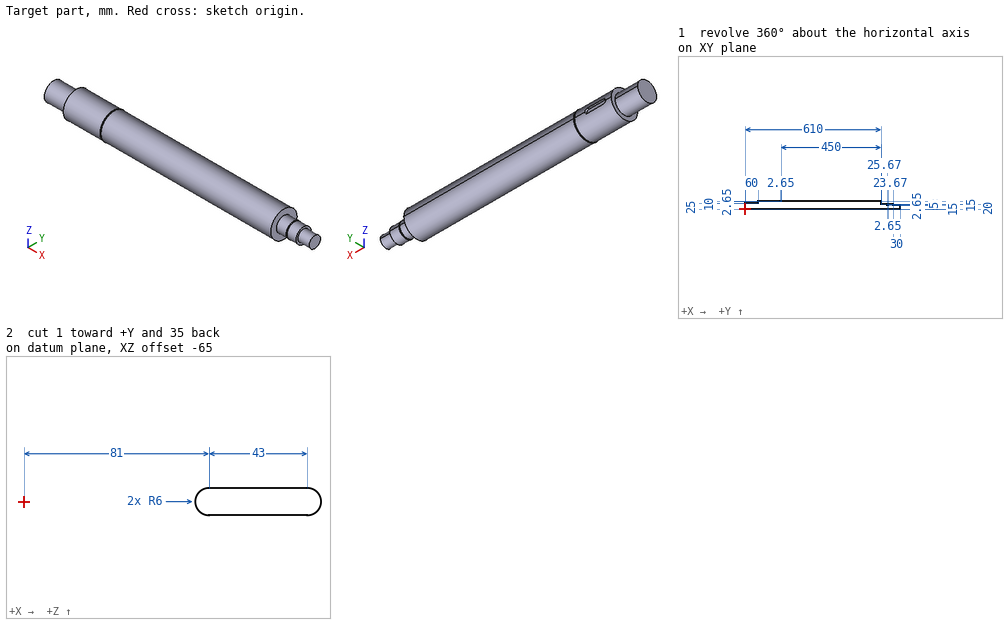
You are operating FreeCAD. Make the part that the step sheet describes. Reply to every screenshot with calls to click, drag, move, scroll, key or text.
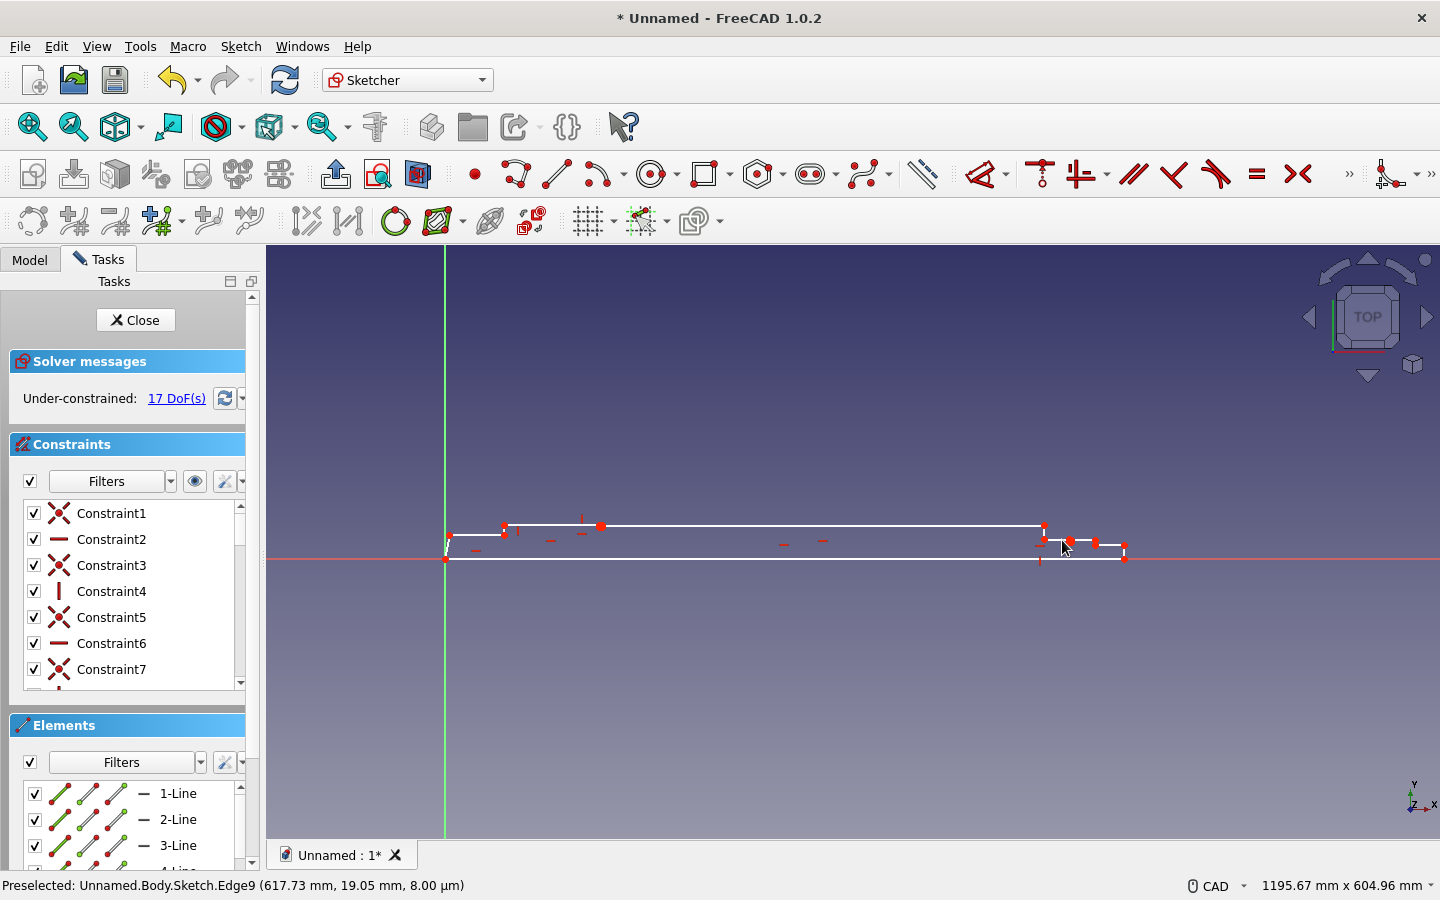
scroll(446, 552, up, 4)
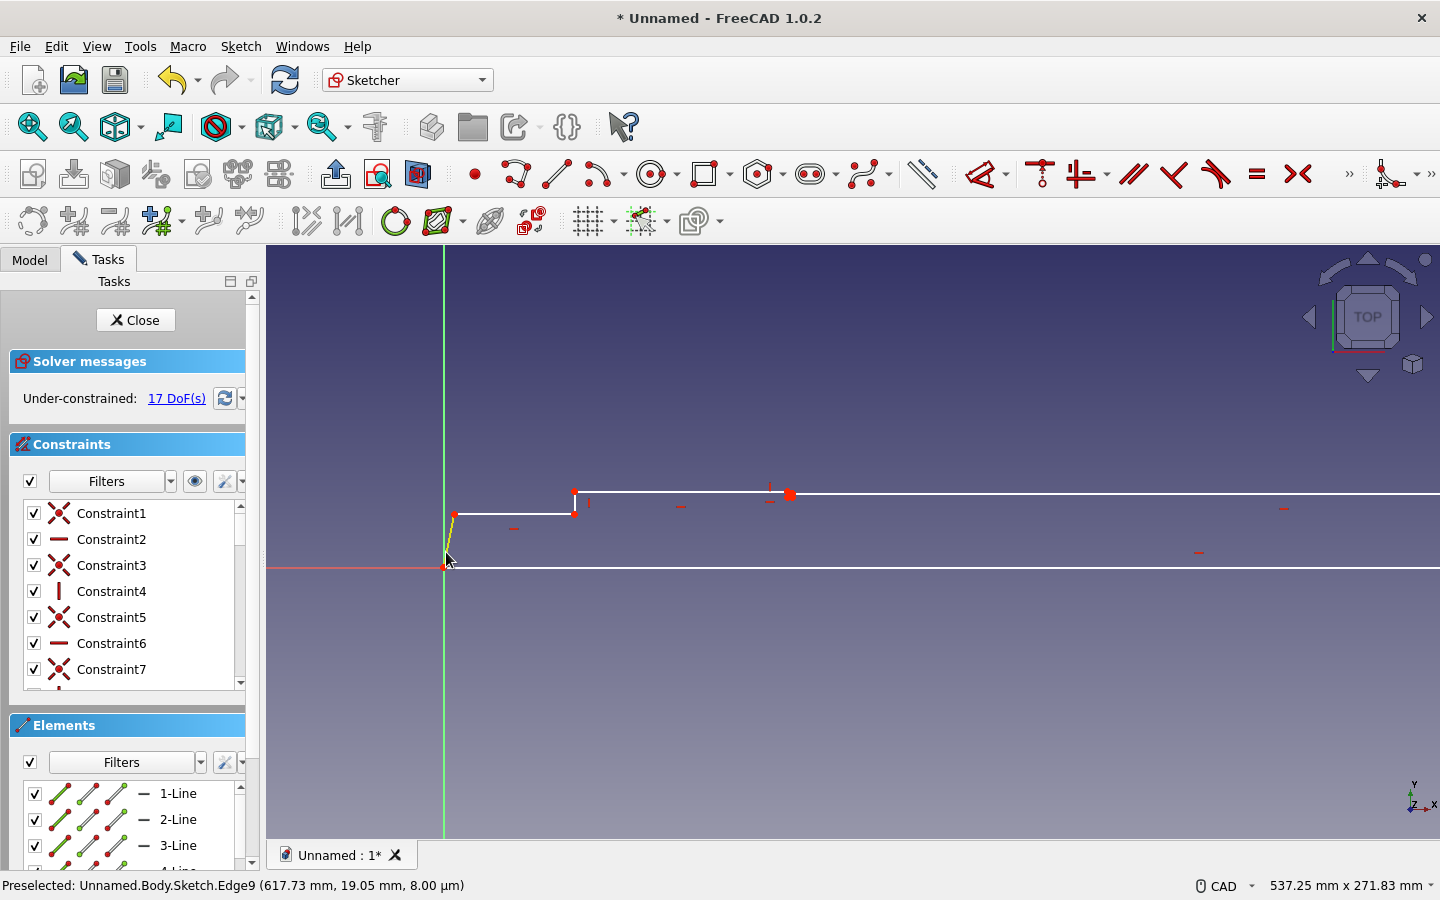
click(447, 552)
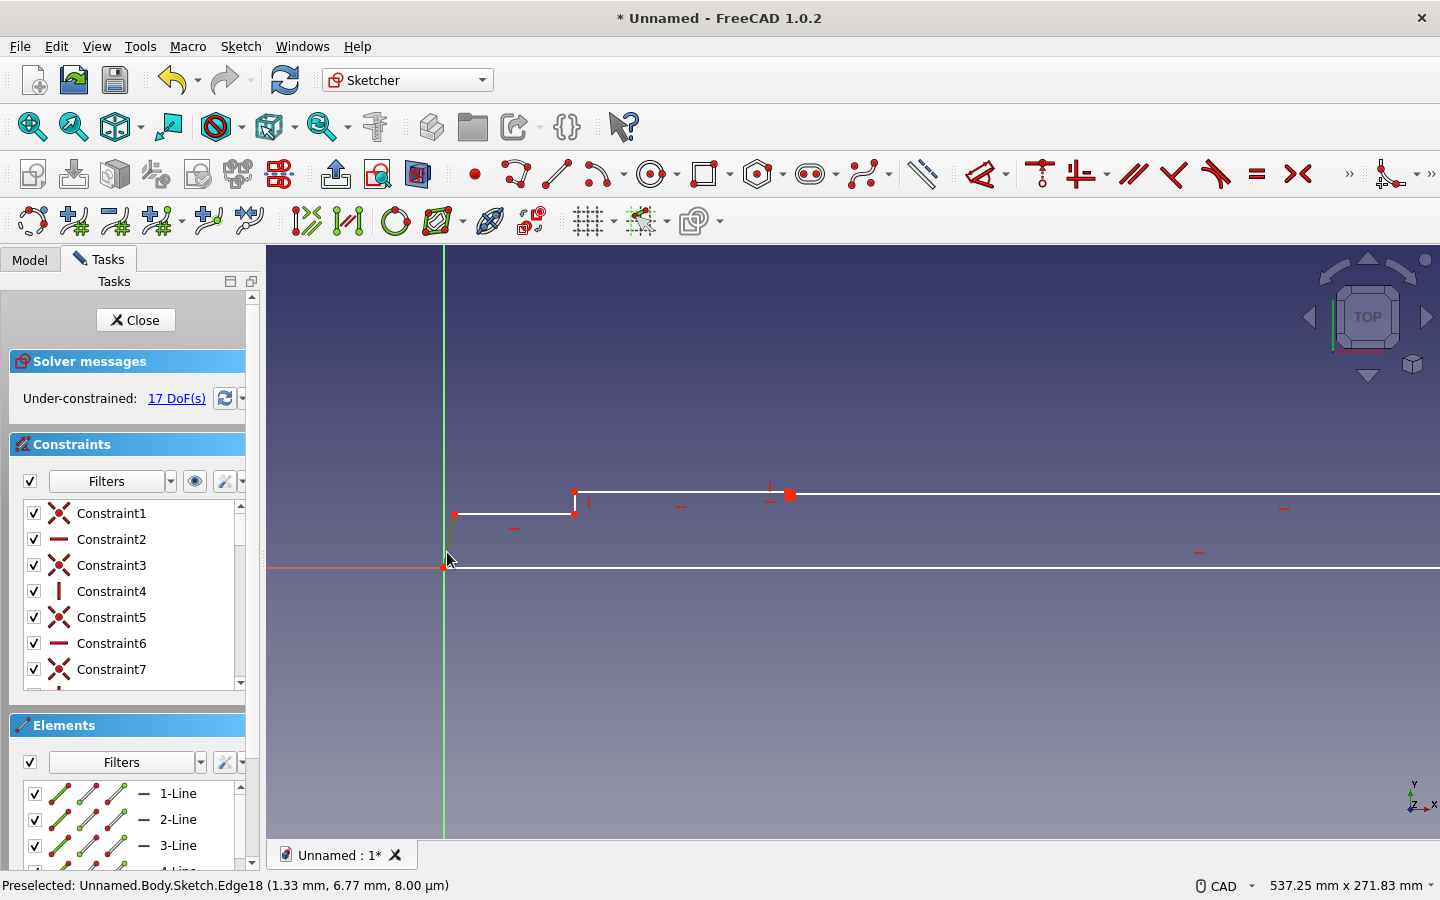
click(1106, 174)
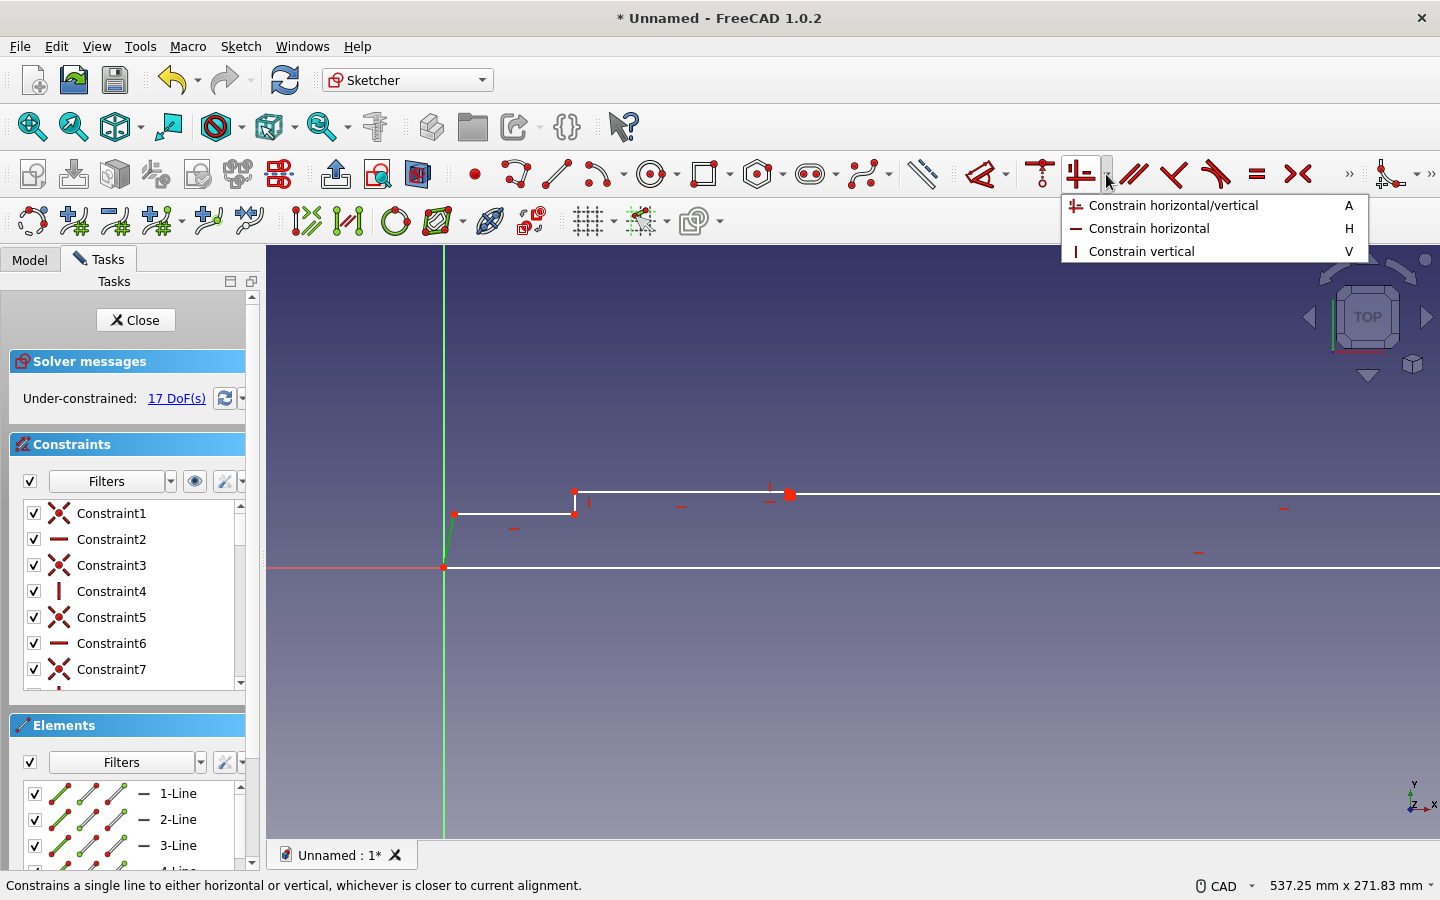
click(1215, 252)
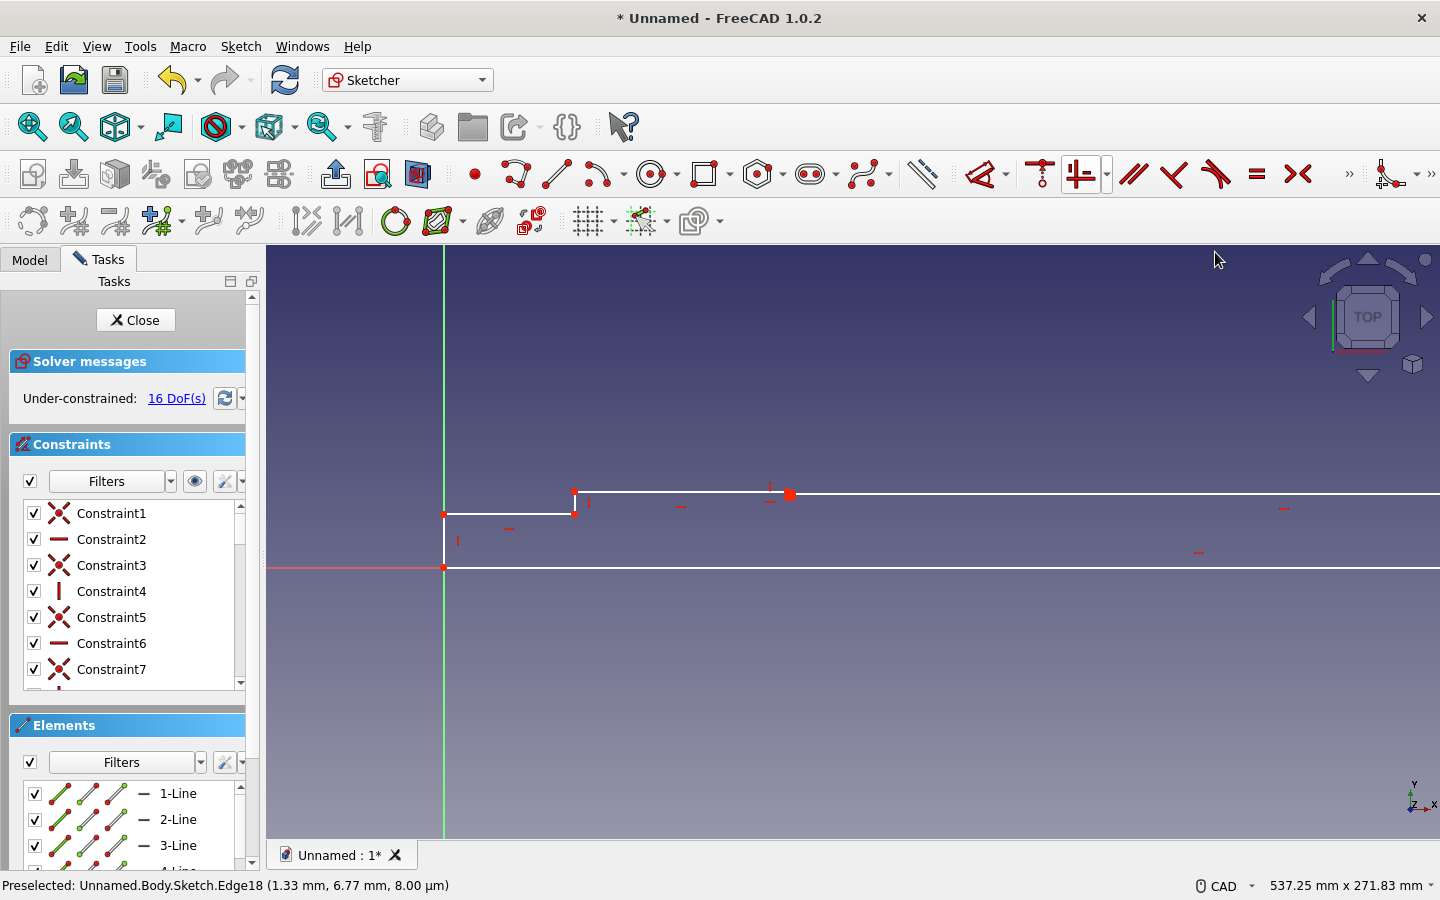
scroll(446, 552, down, 4)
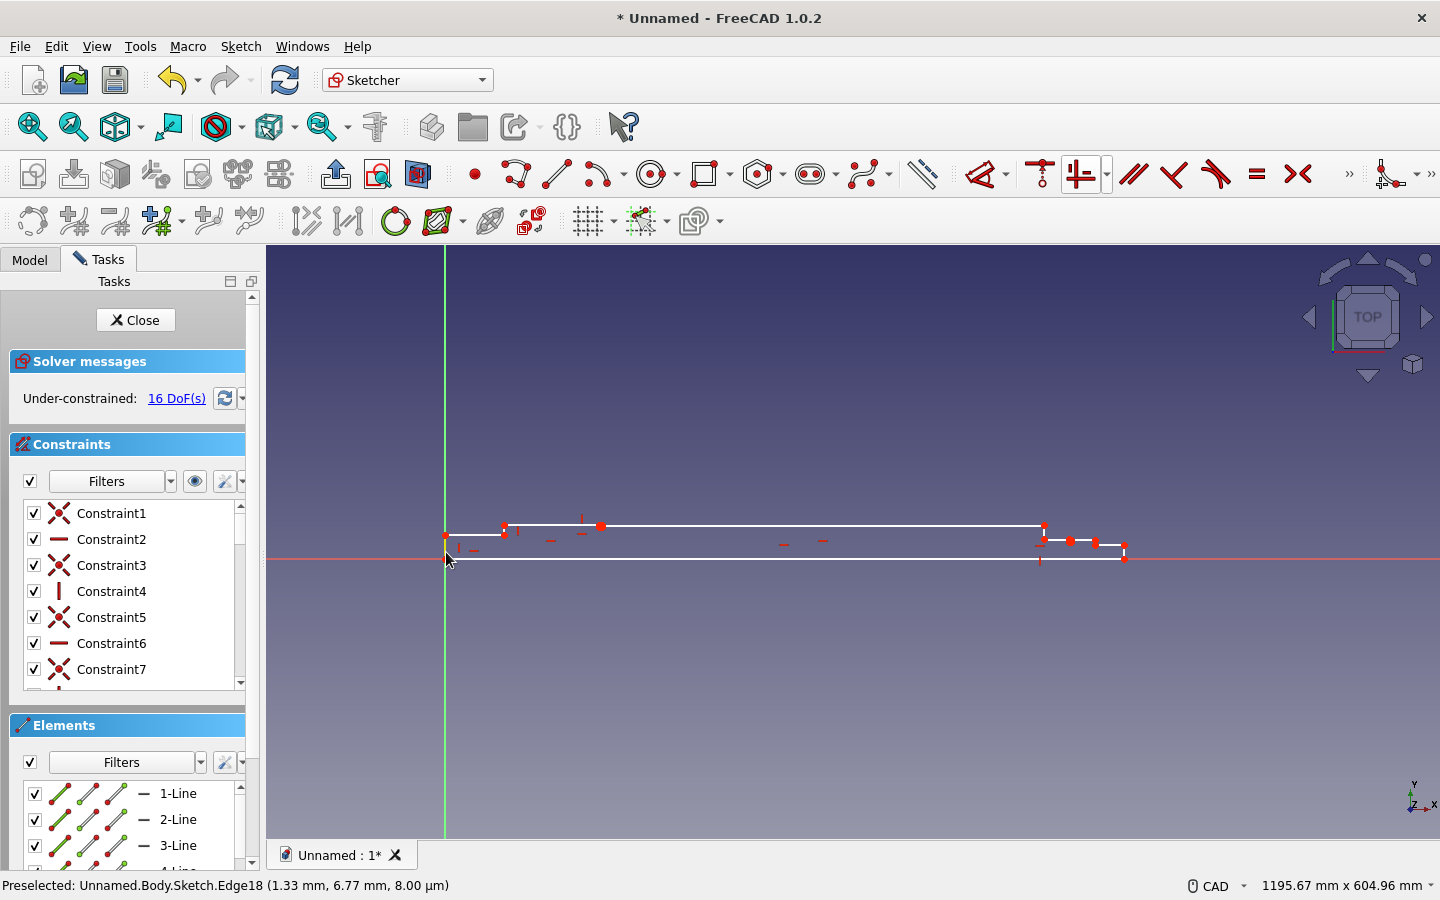
scroll(1095, 543, up, 11)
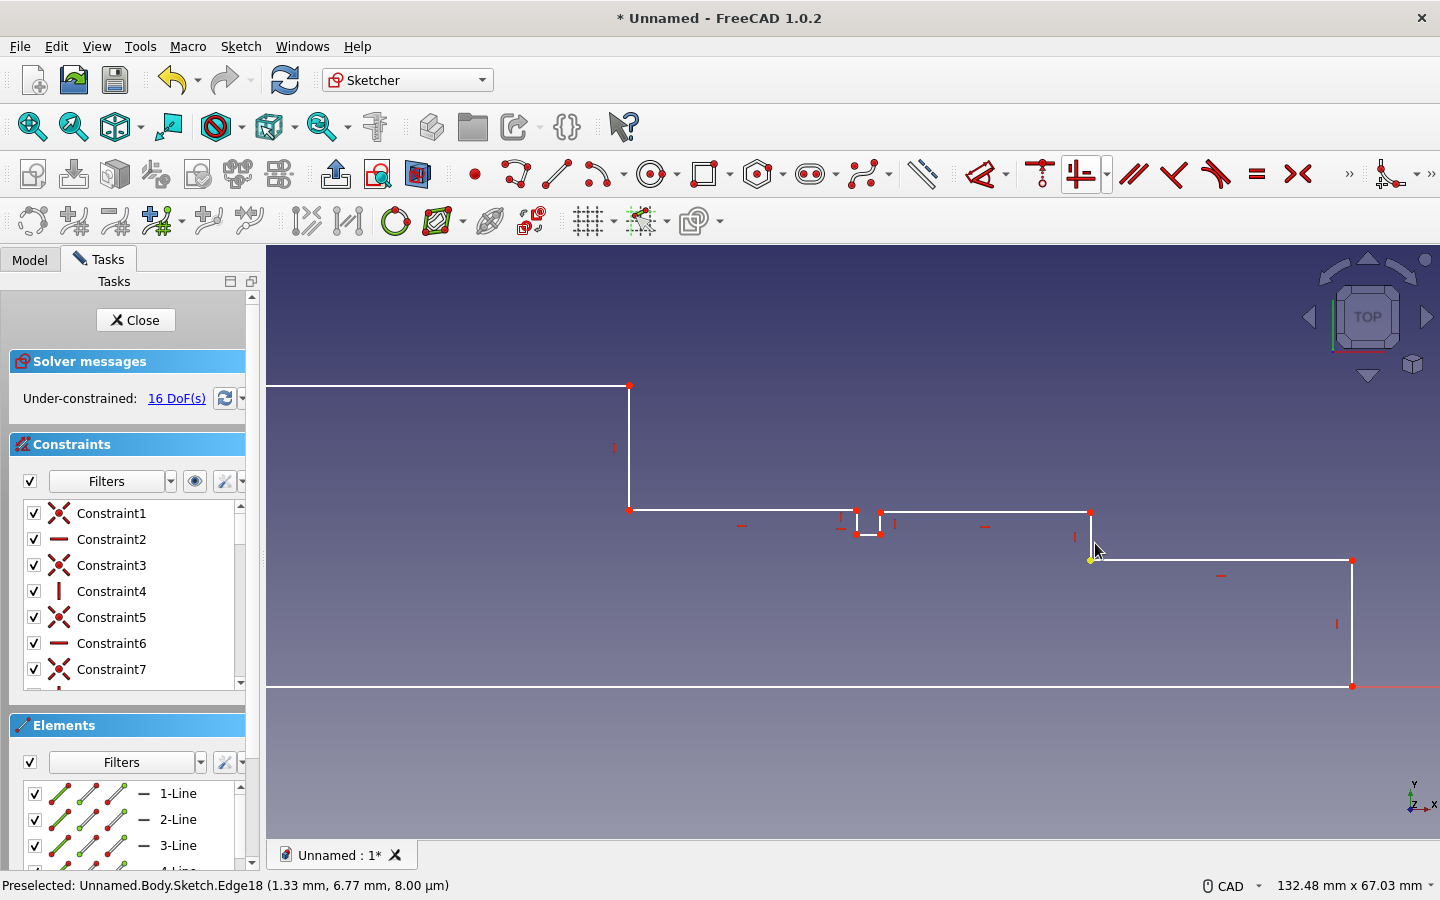
click(1091, 536)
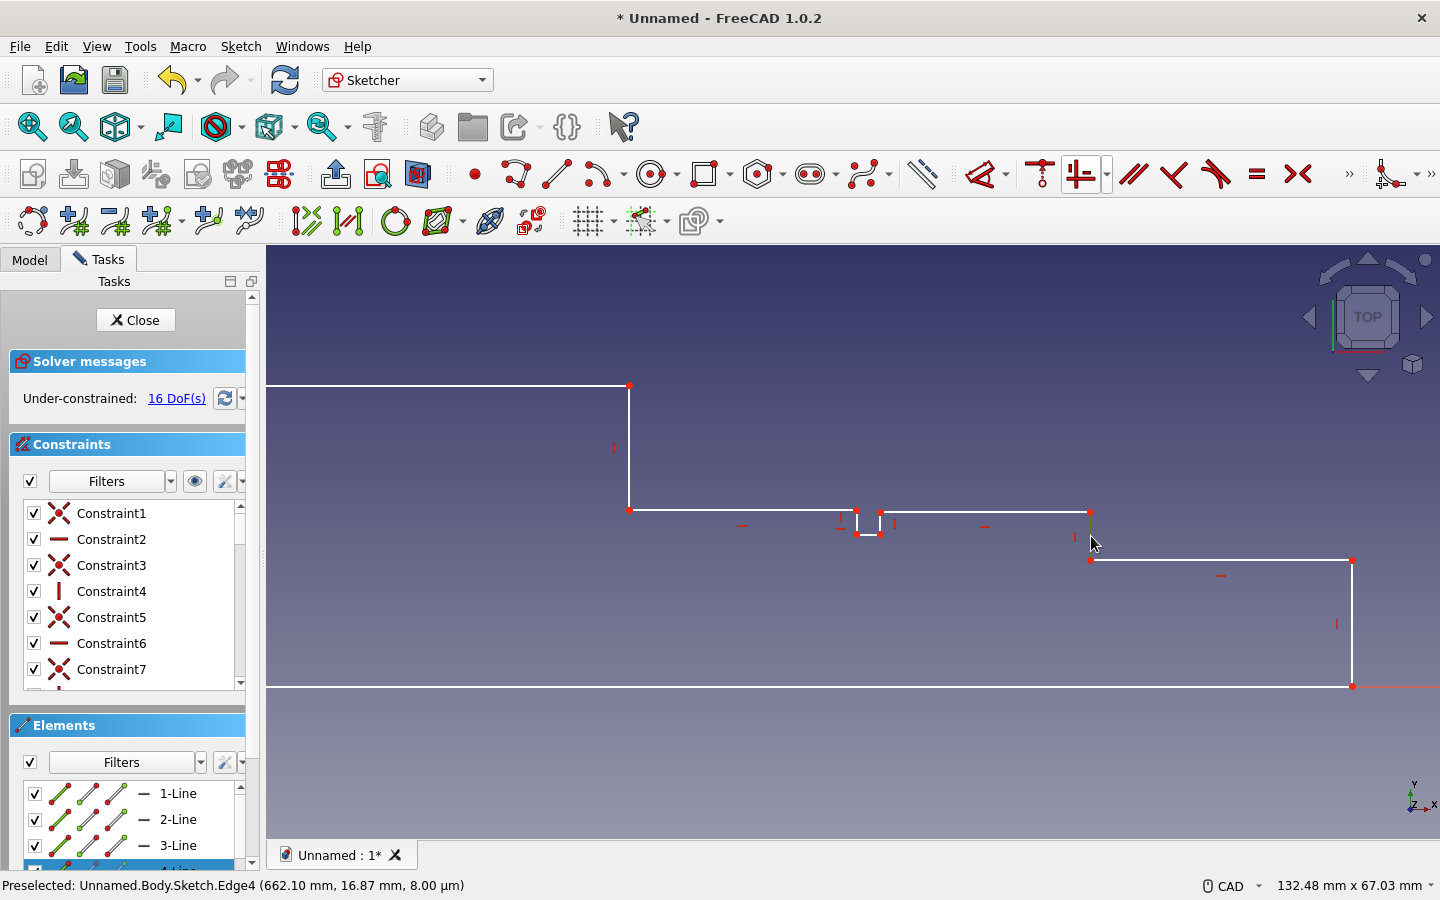
click(1006, 174)